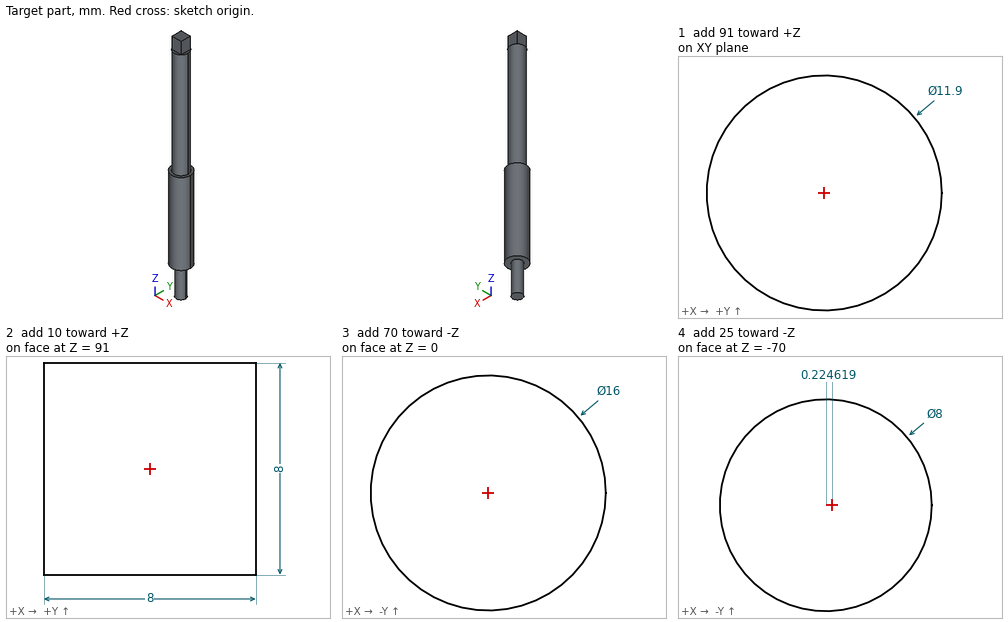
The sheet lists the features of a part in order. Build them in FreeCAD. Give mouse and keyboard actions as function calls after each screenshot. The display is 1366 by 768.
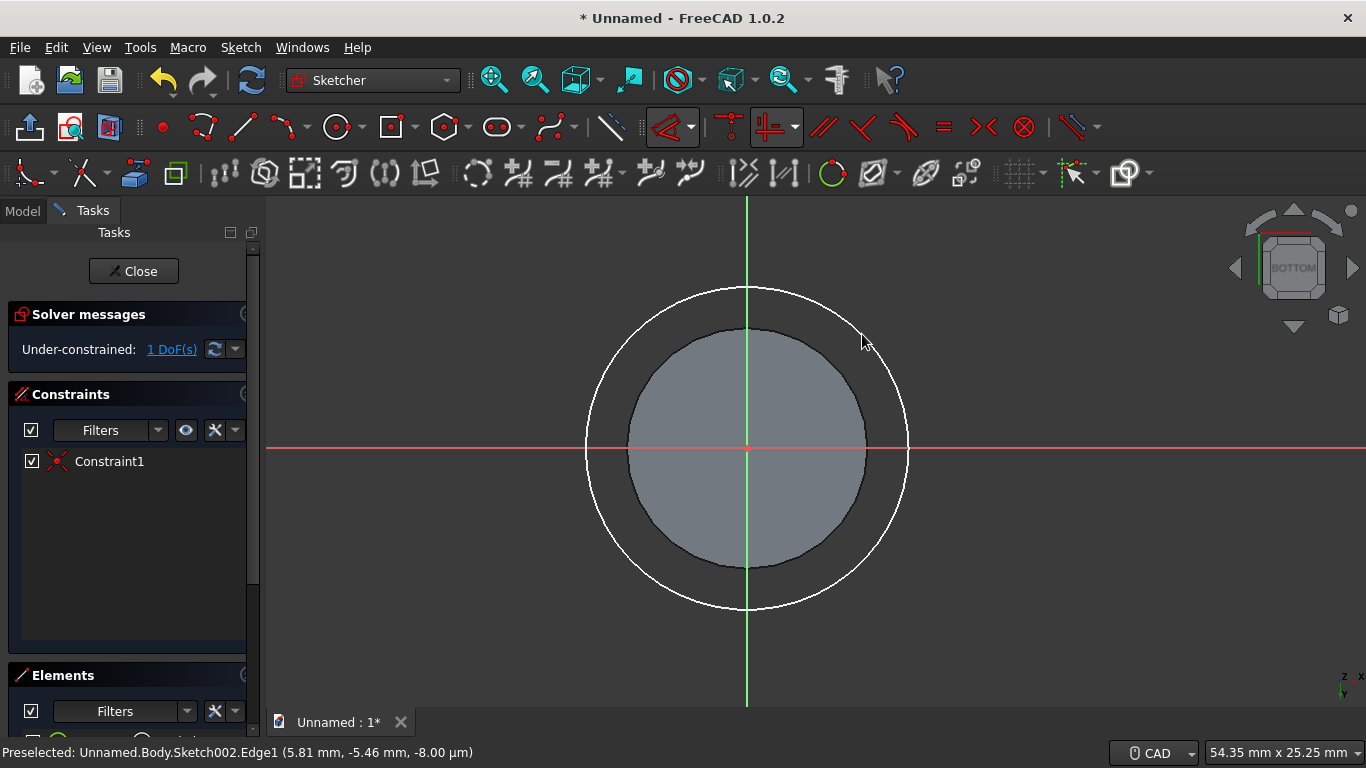
click(861, 334)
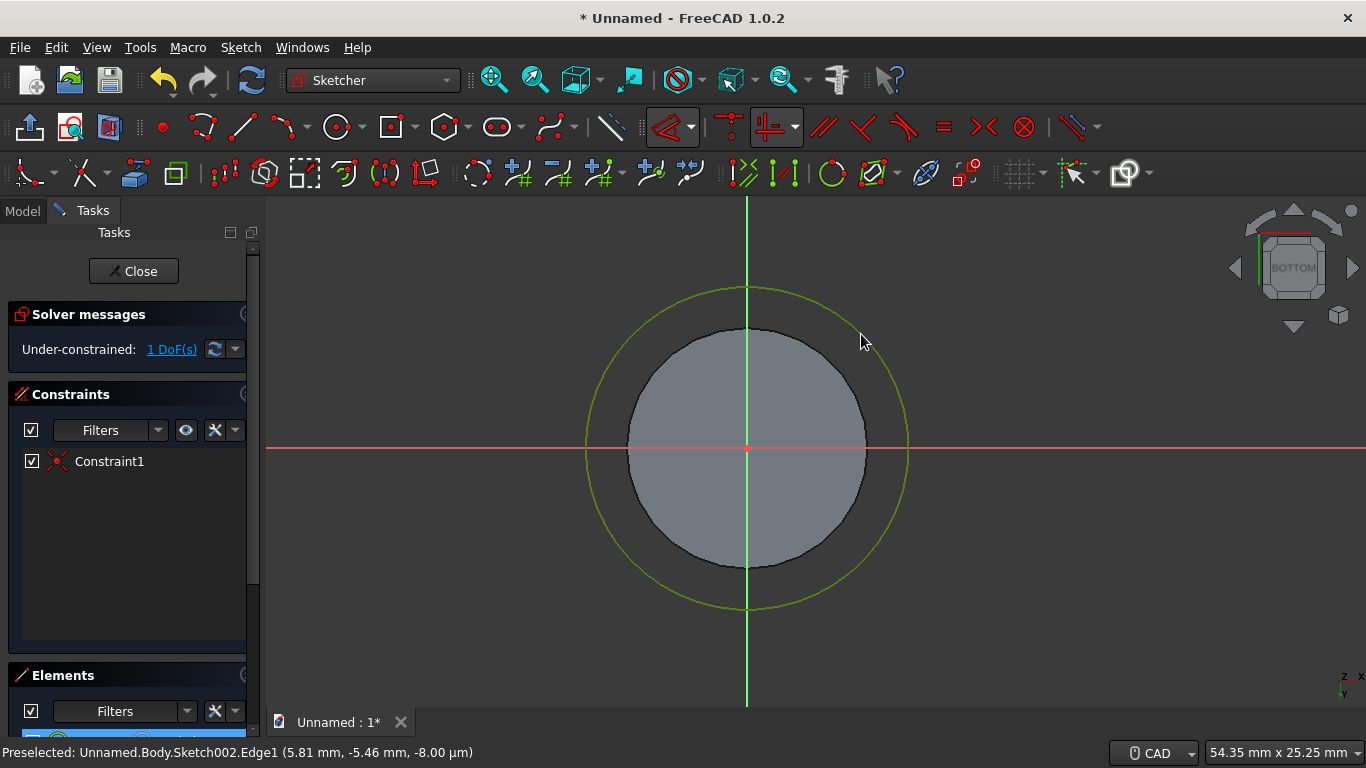
key(k)
key(o)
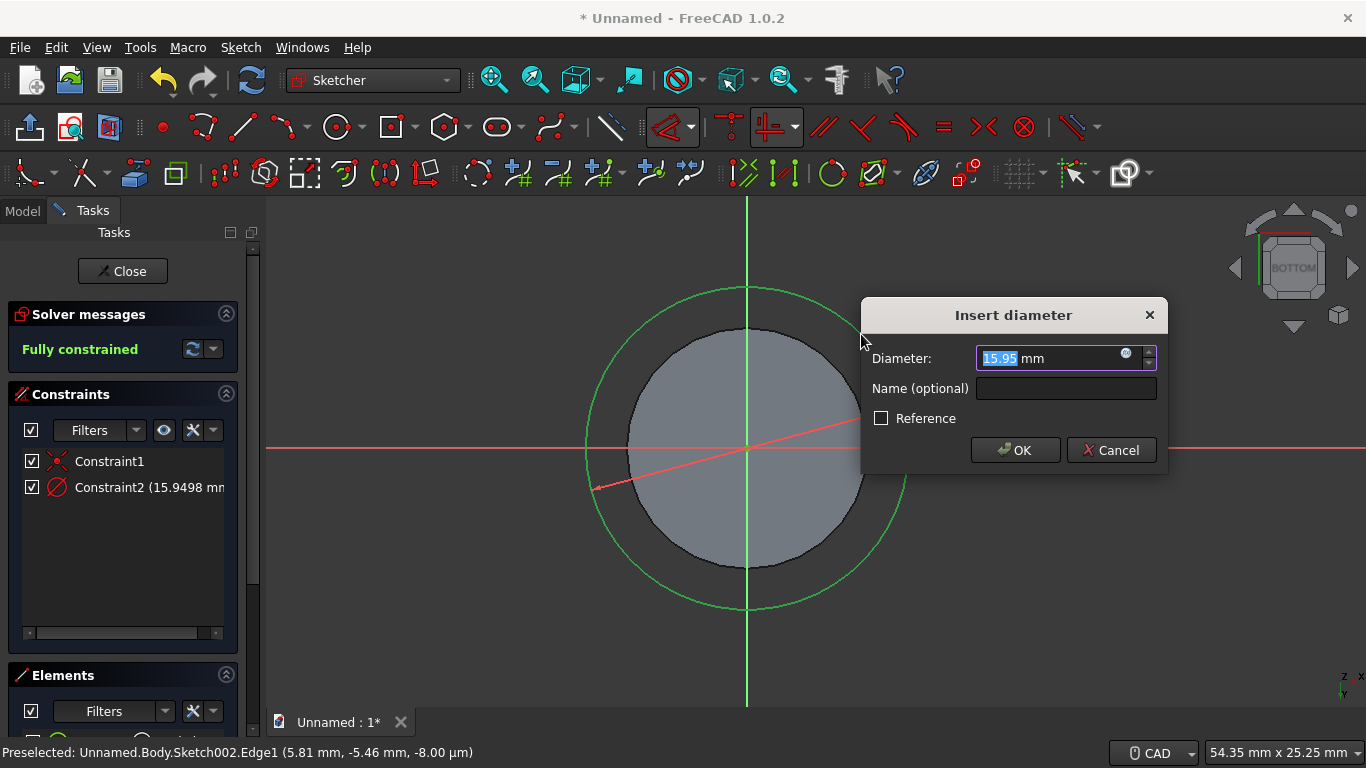
text(16)
key(Return)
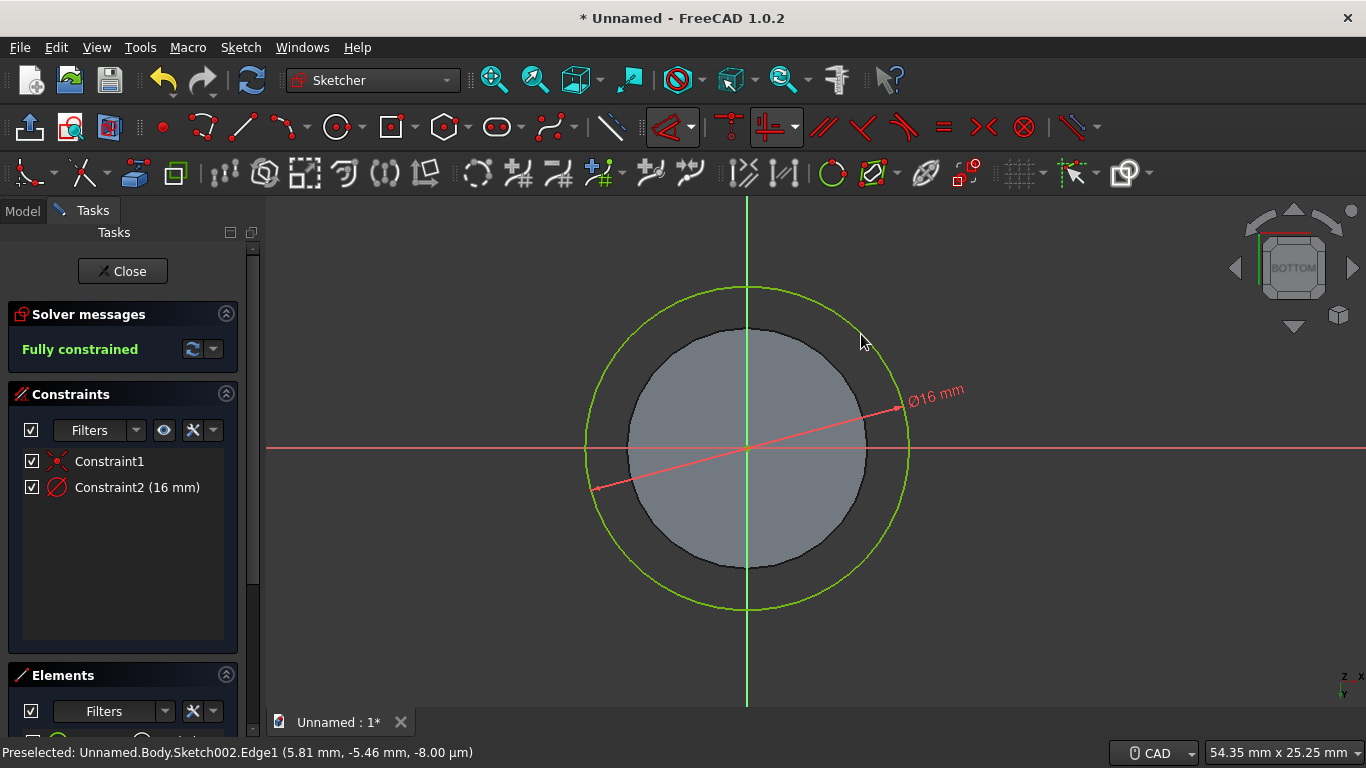
click(123, 271)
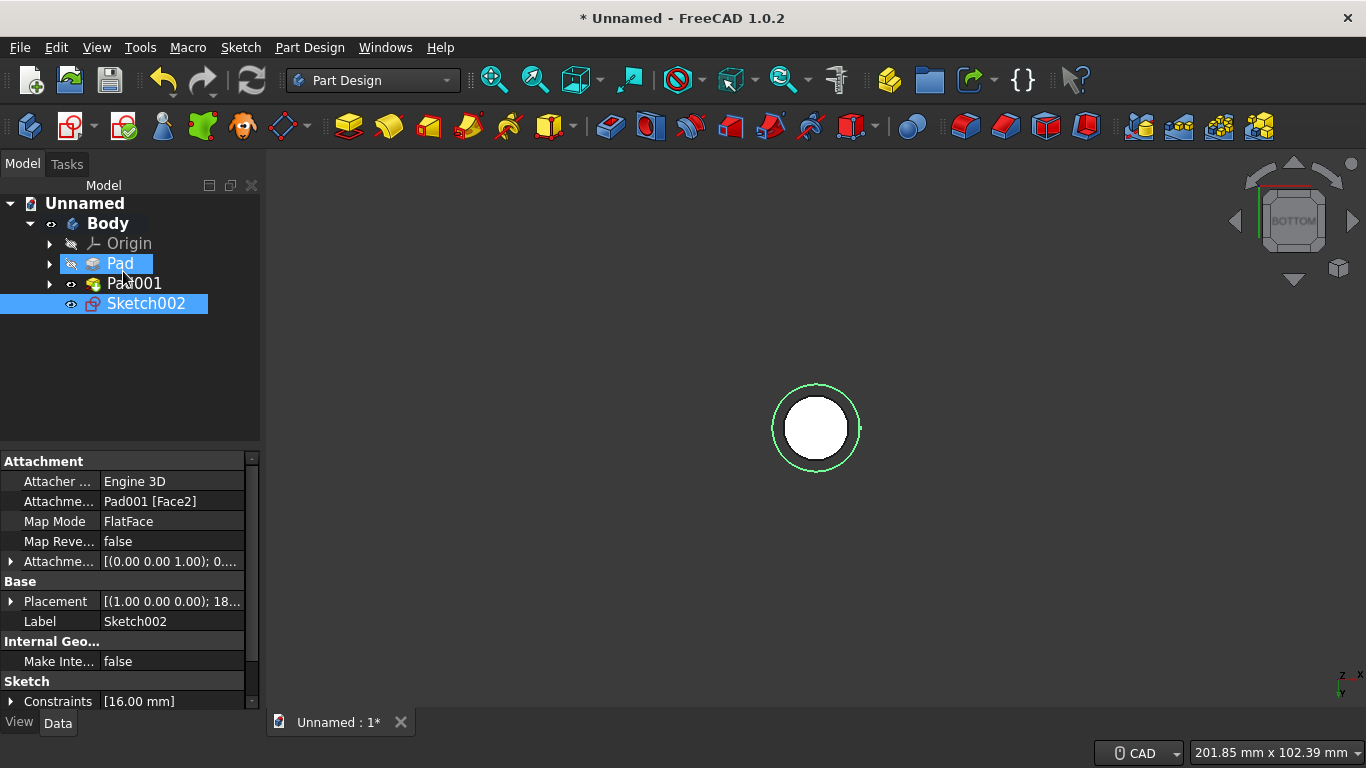
click(350, 126)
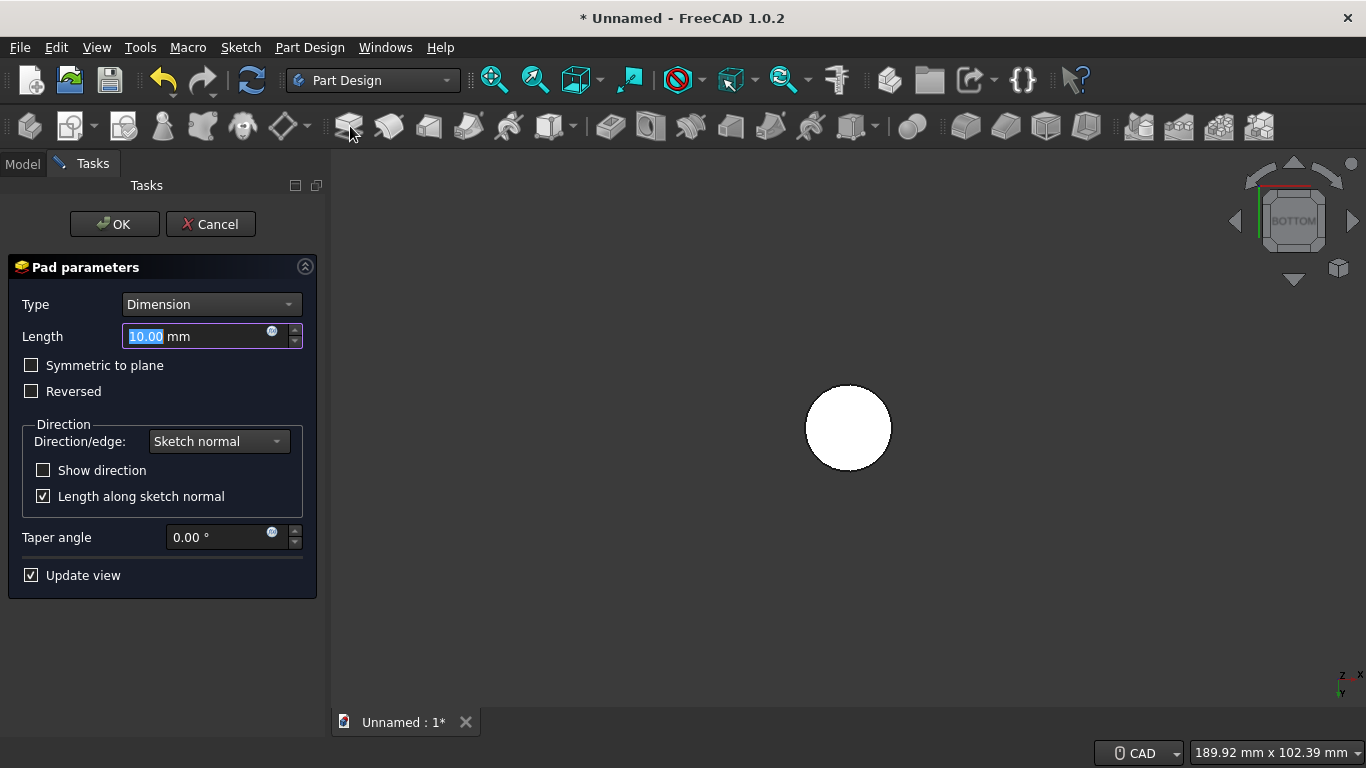
text(70)
key(Tab)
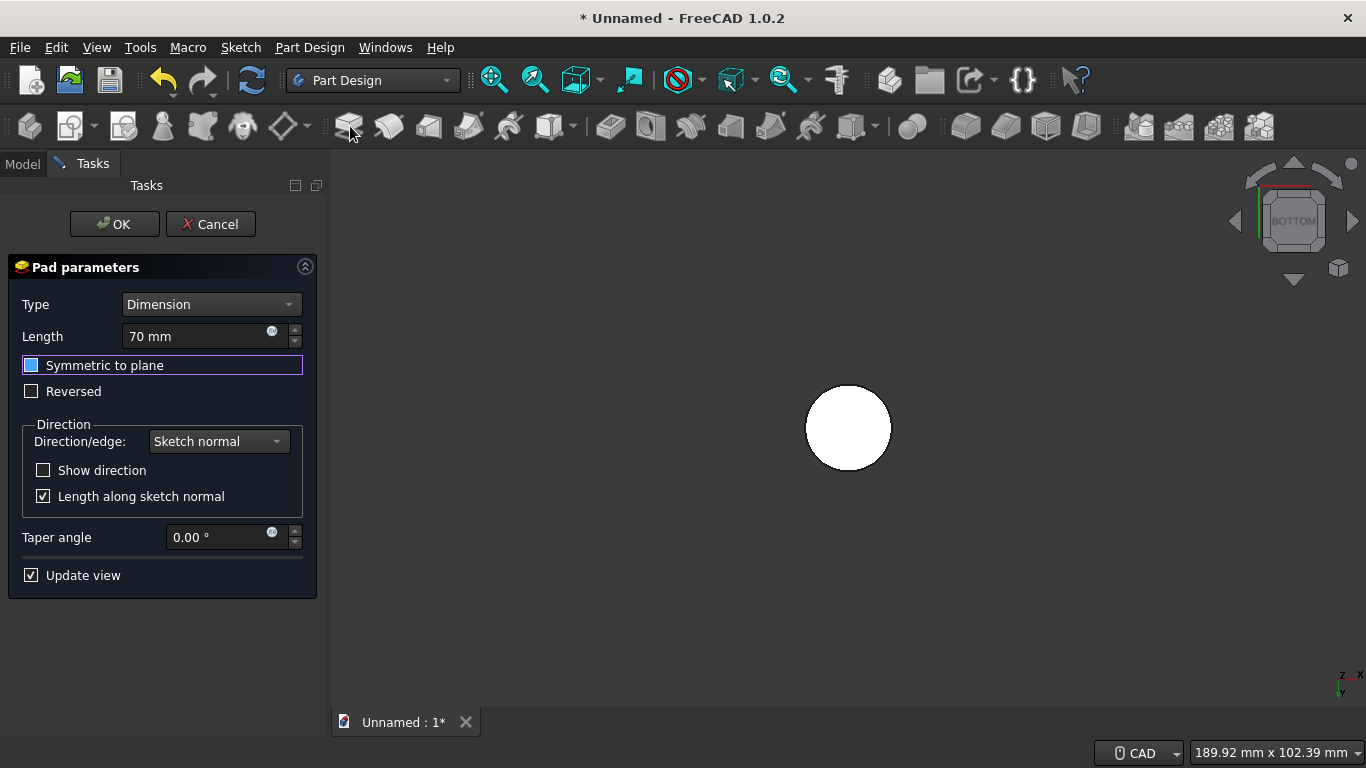
click(115, 224)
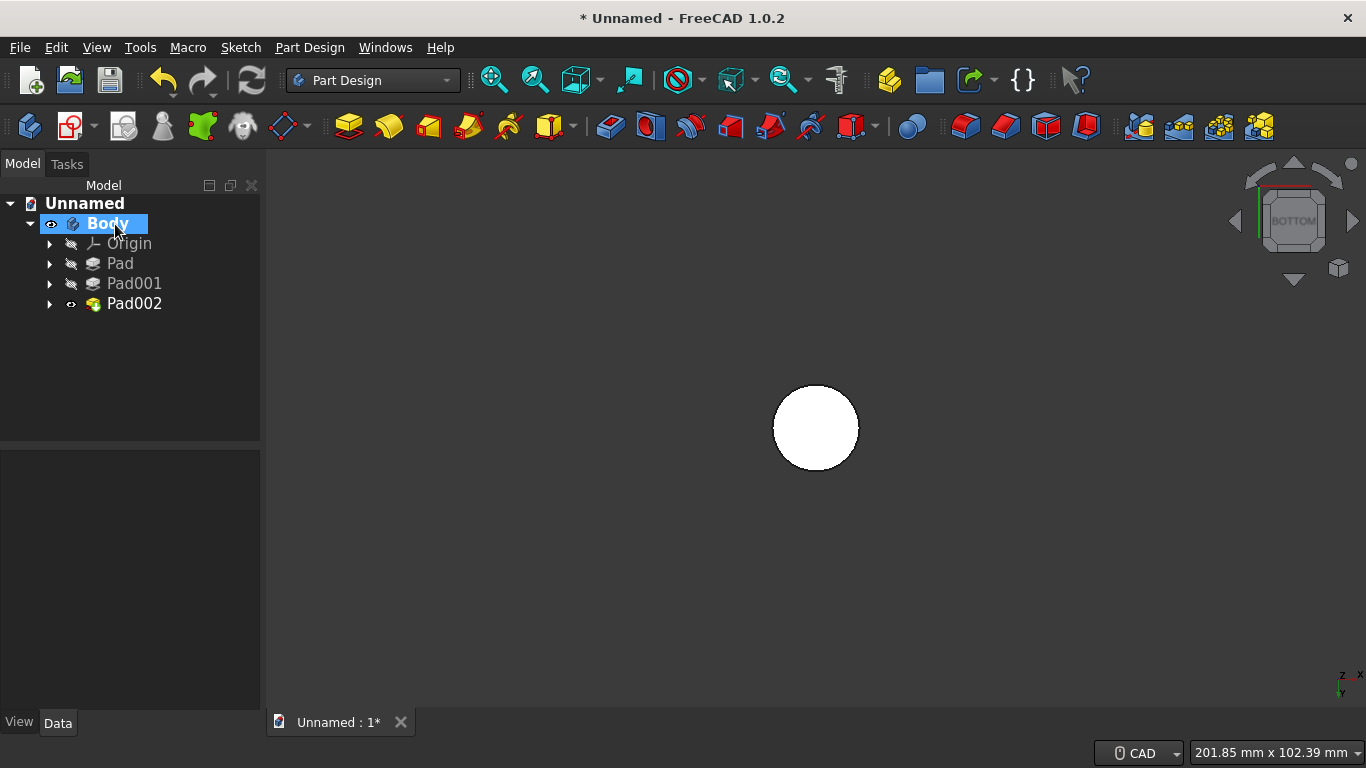
click(496, 80)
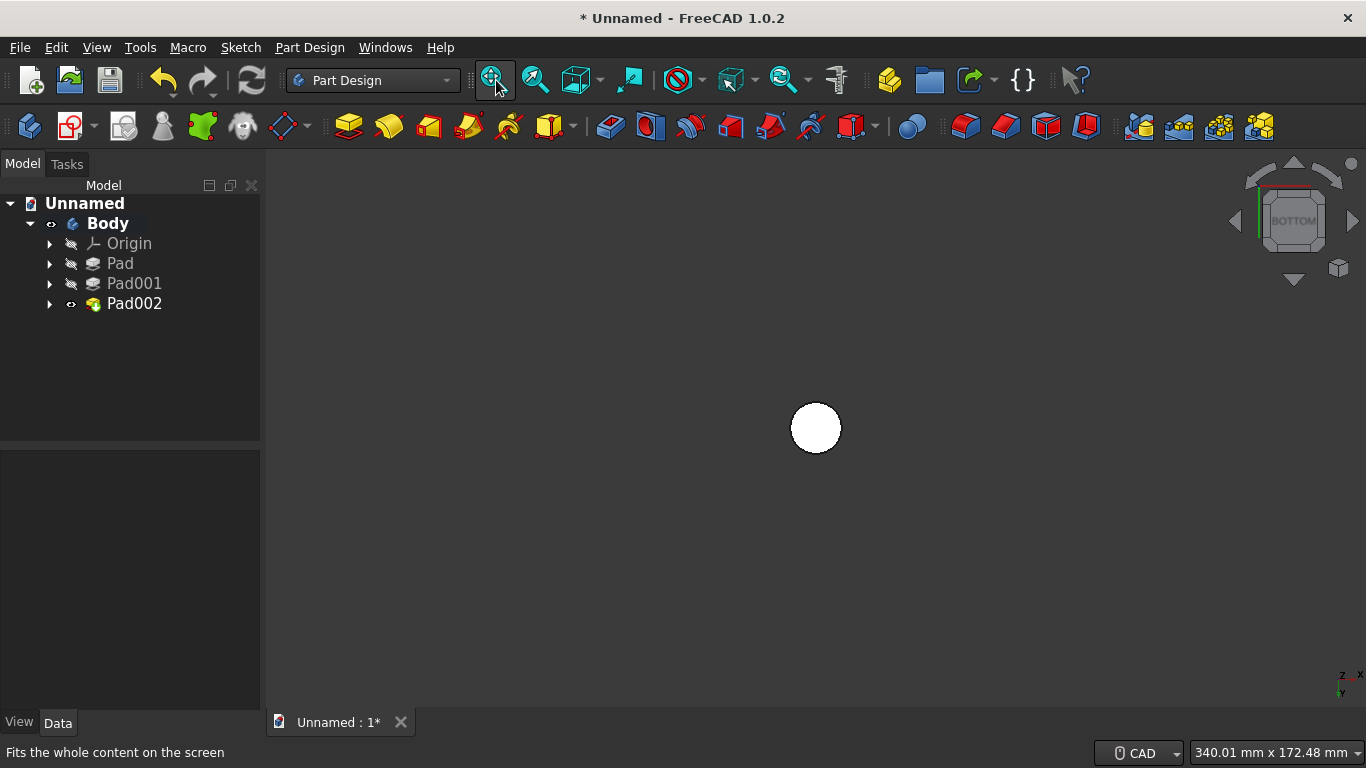
click(816, 427)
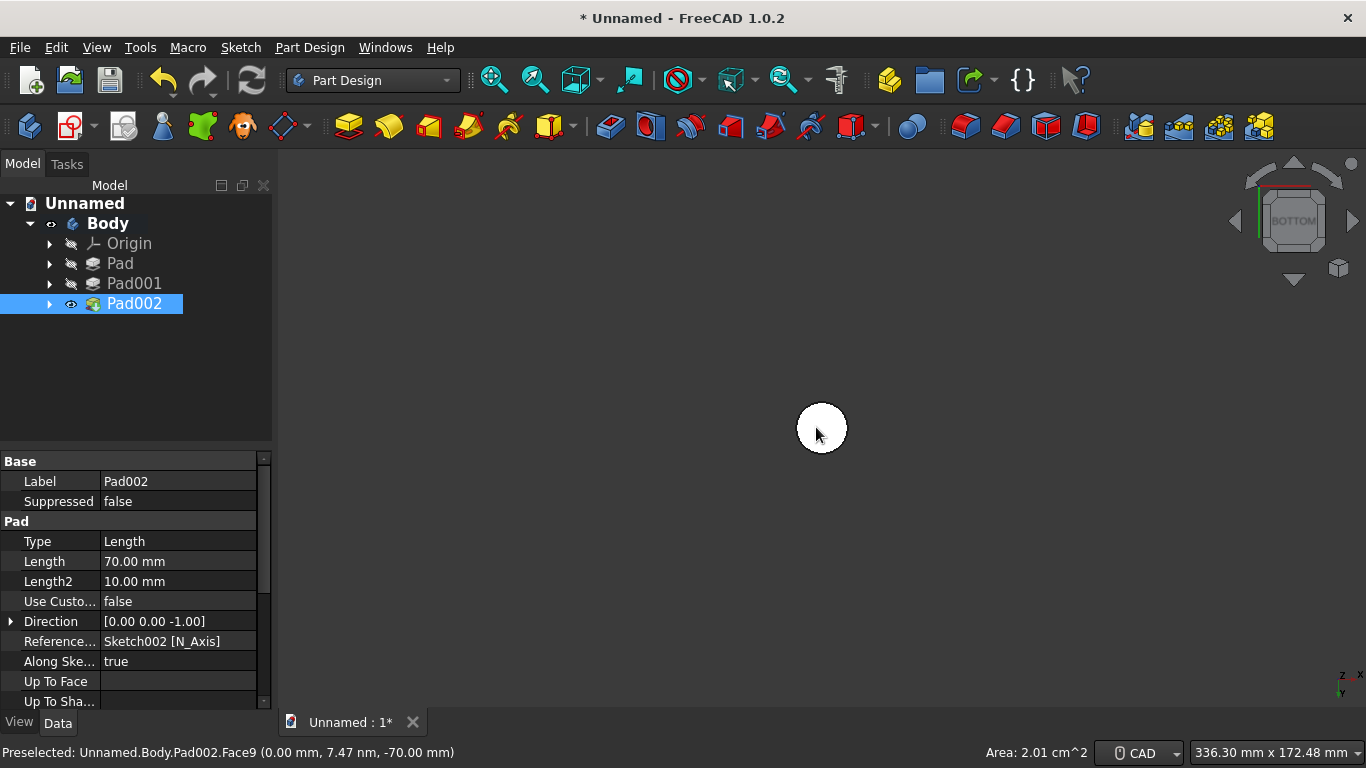
click(70, 126)